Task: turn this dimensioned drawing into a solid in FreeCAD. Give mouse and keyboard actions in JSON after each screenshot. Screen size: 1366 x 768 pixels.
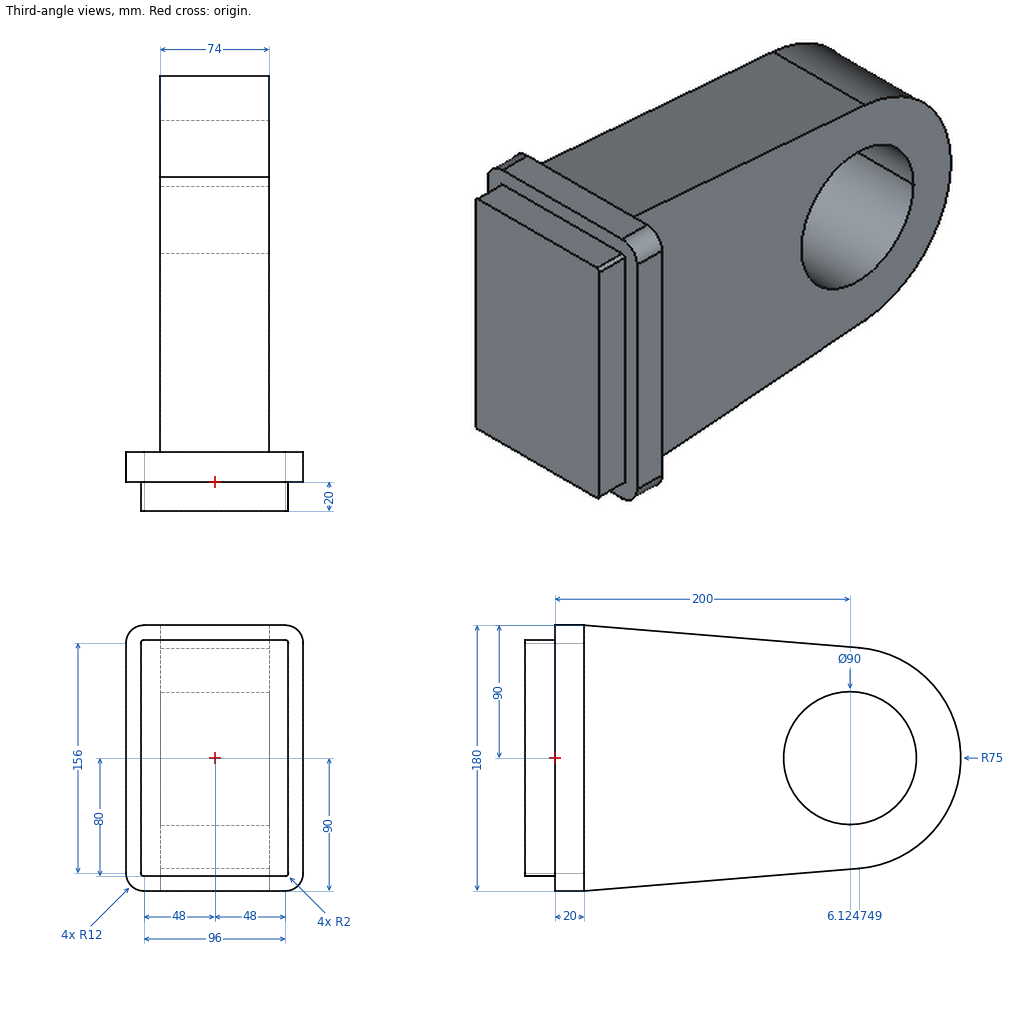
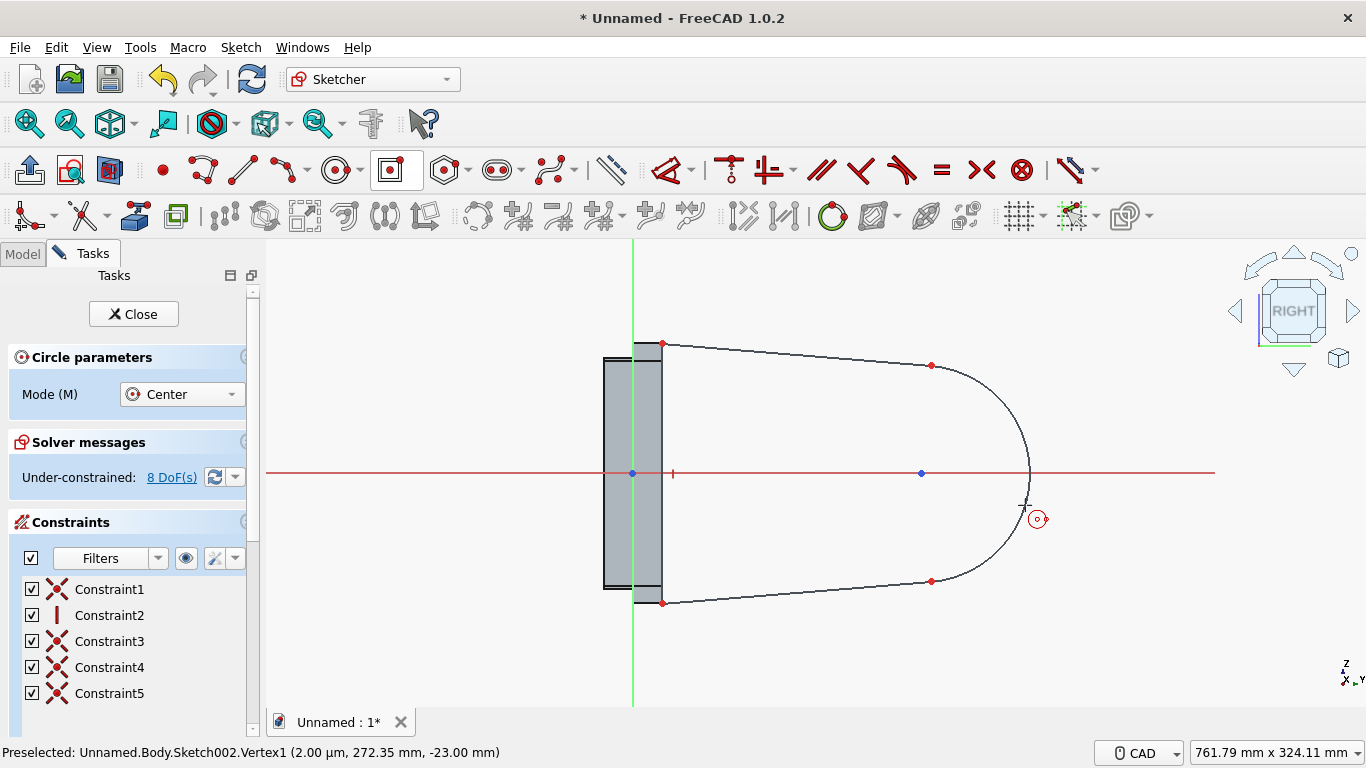
{"action": "left_click", "coordinate": [922, 473]}
{"action": "mouse_move", "coordinate": [968, 427]}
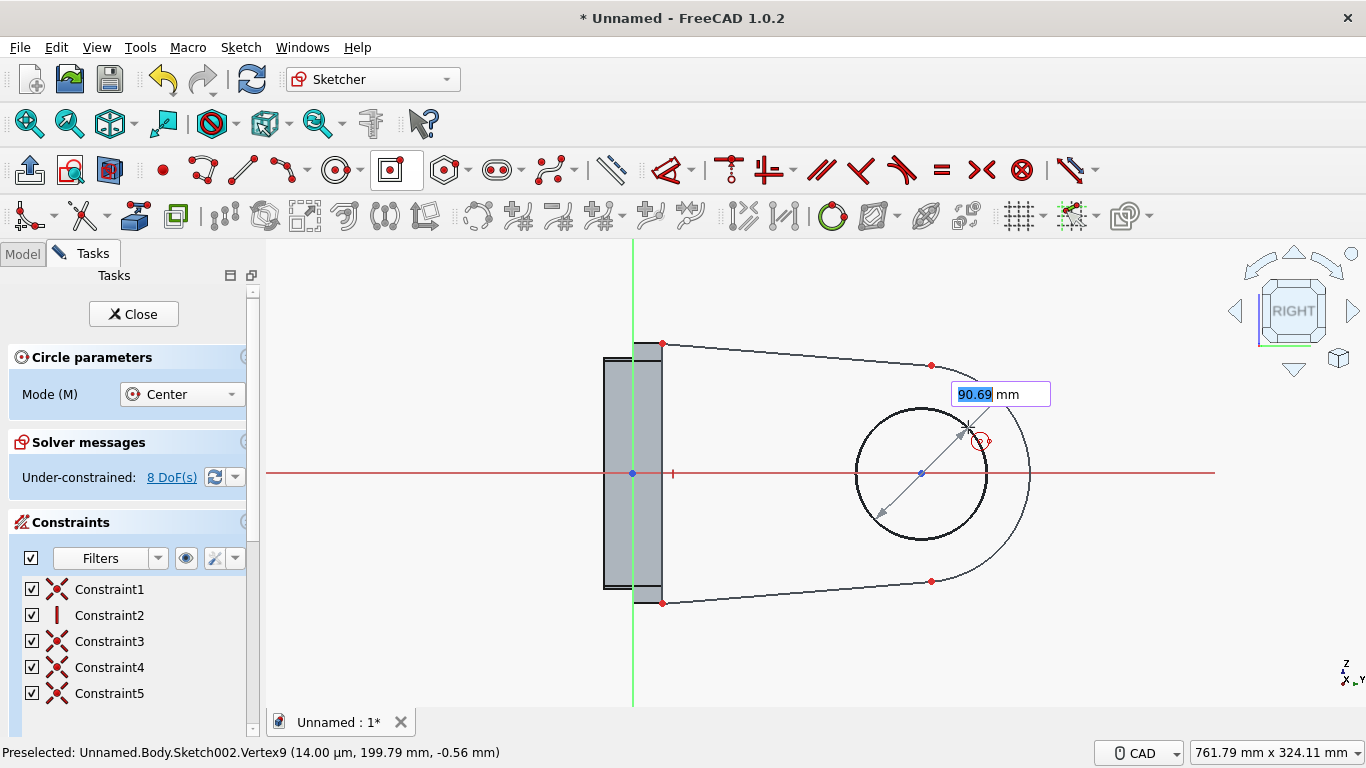
{"action": "type", "text": "90"}
{"action": "key", "text": "Return"}
{"action": "key", "text": "Escape"}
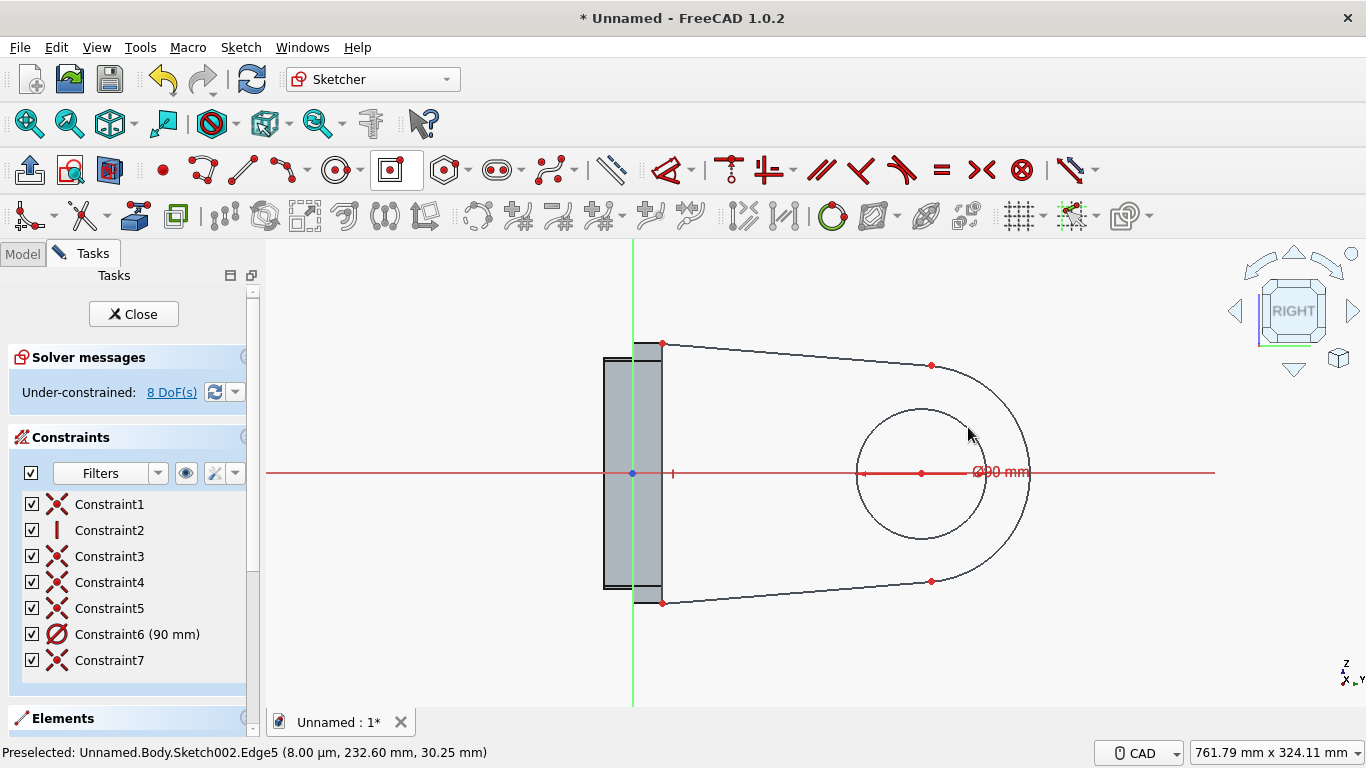
{"action": "left_click", "coordinate": [921, 474]}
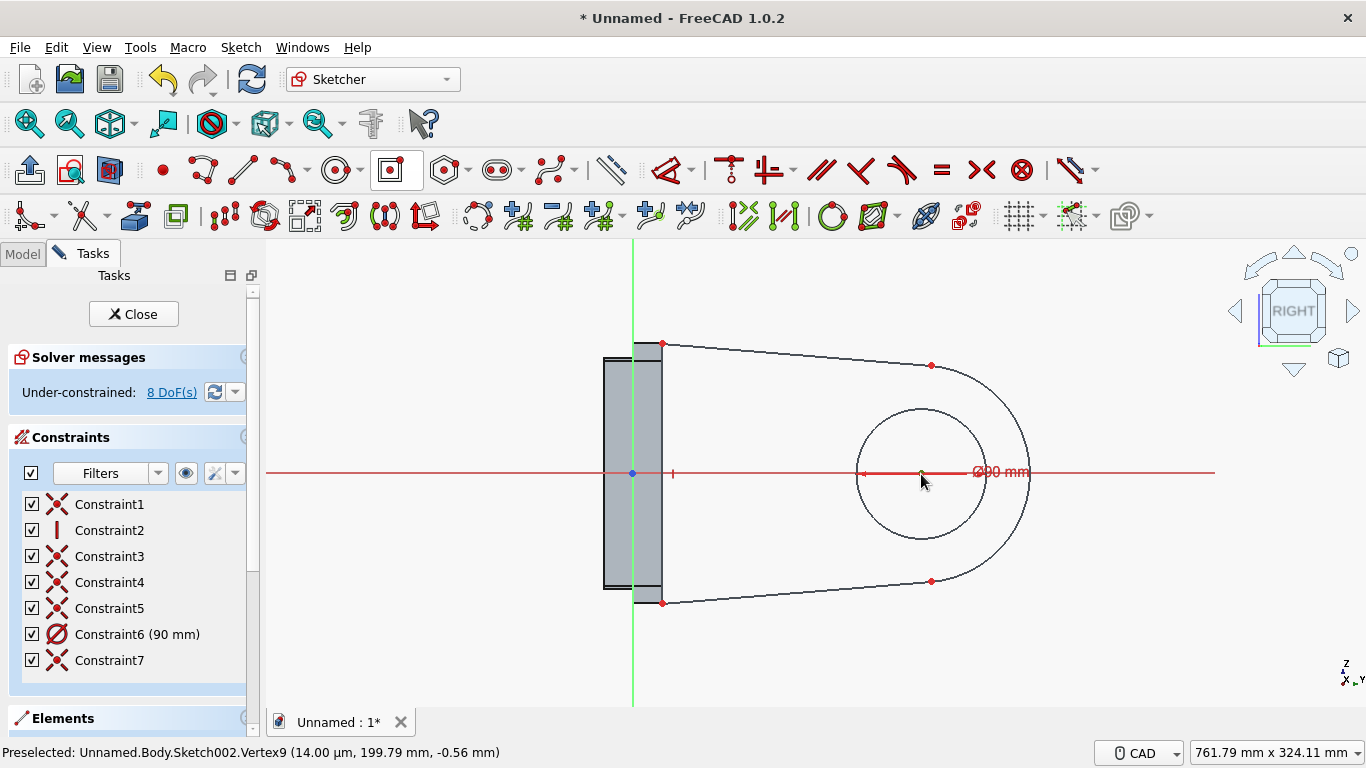
{"action": "left_click", "coordinate": [359, 473]}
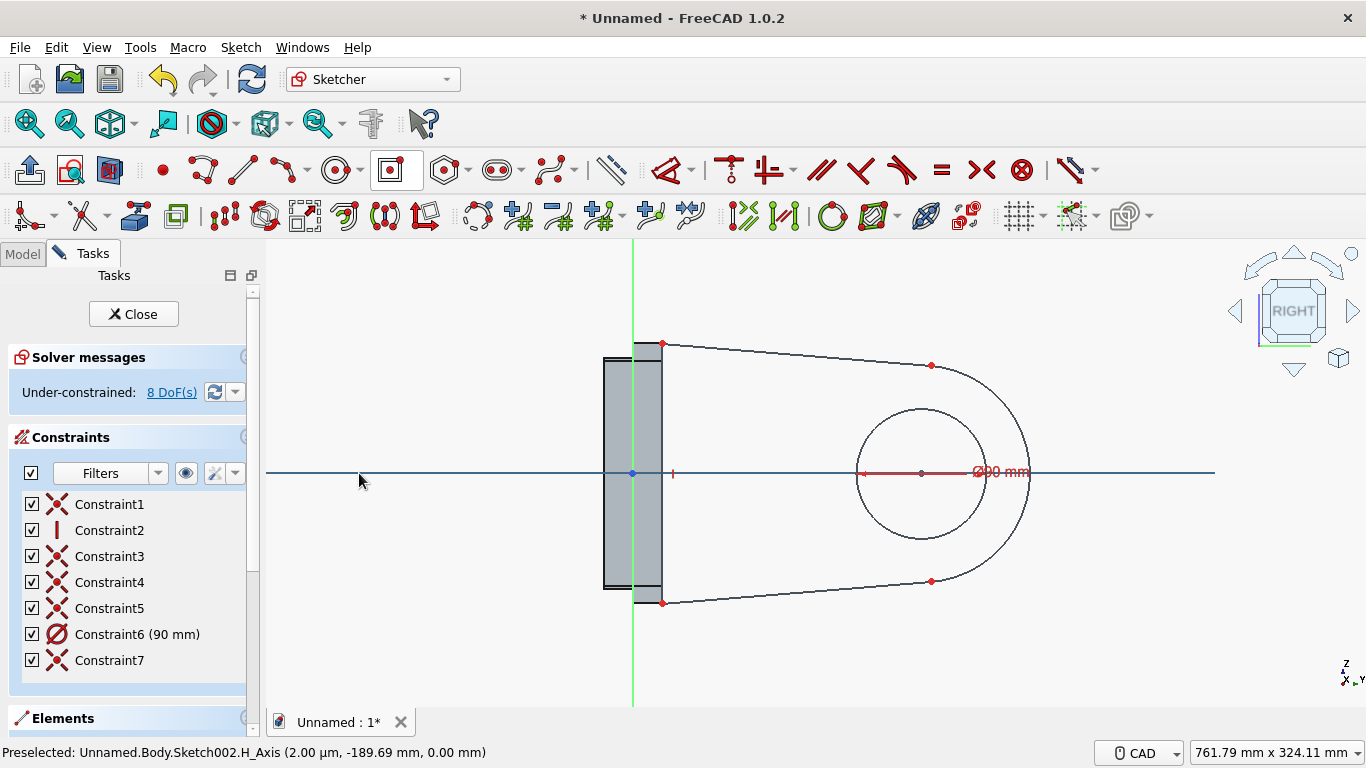
{"action": "left_click", "coordinate": [730, 170]}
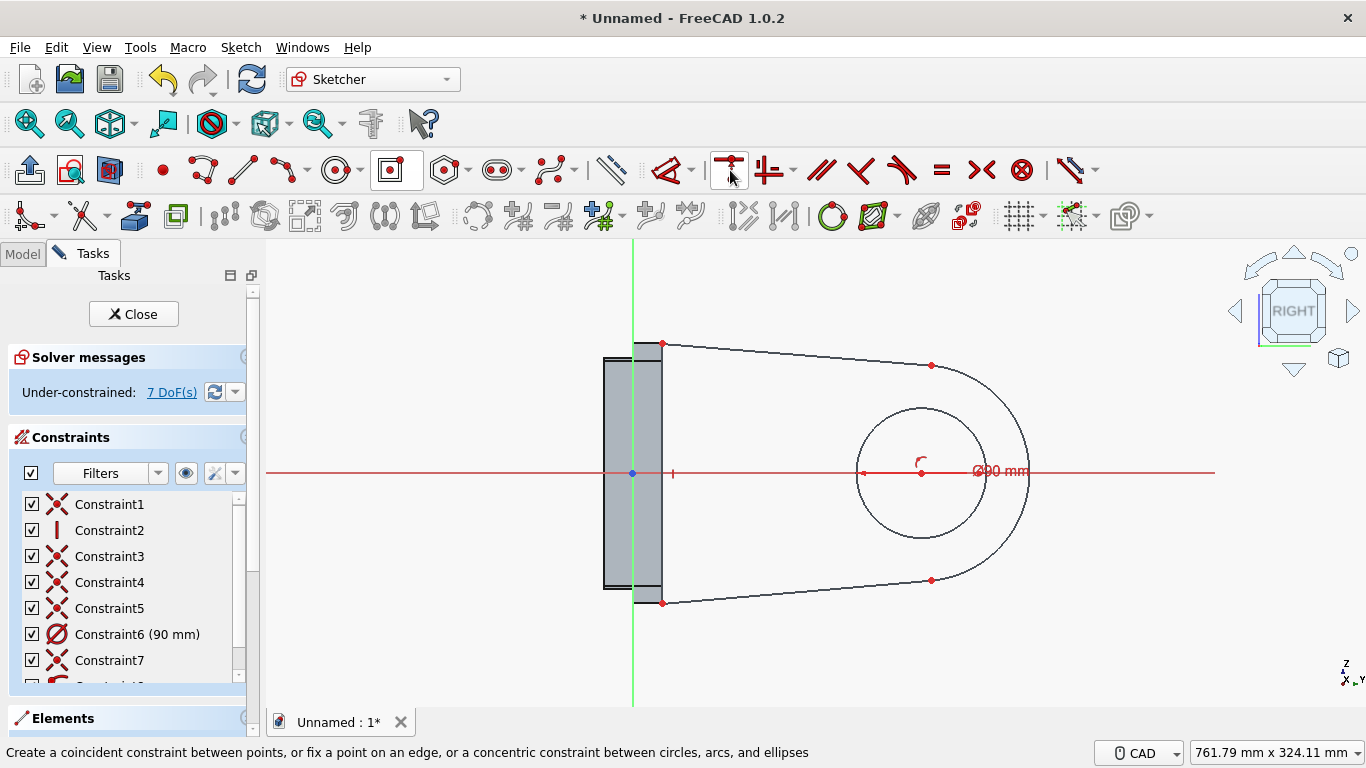
{"action": "key", "text": "d"}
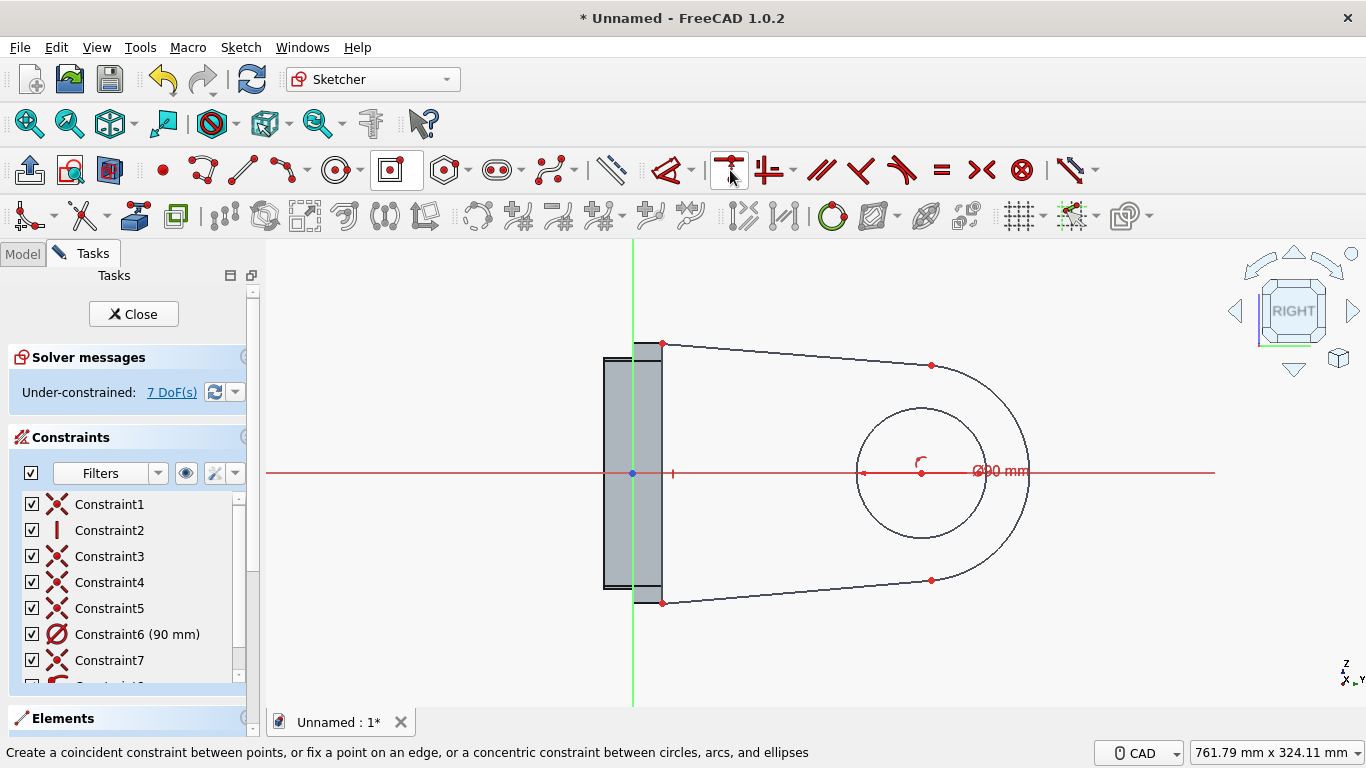
{"action": "left_click", "coordinate": [1011, 534]}
{"action": "left_click", "coordinate": [1037, 552]}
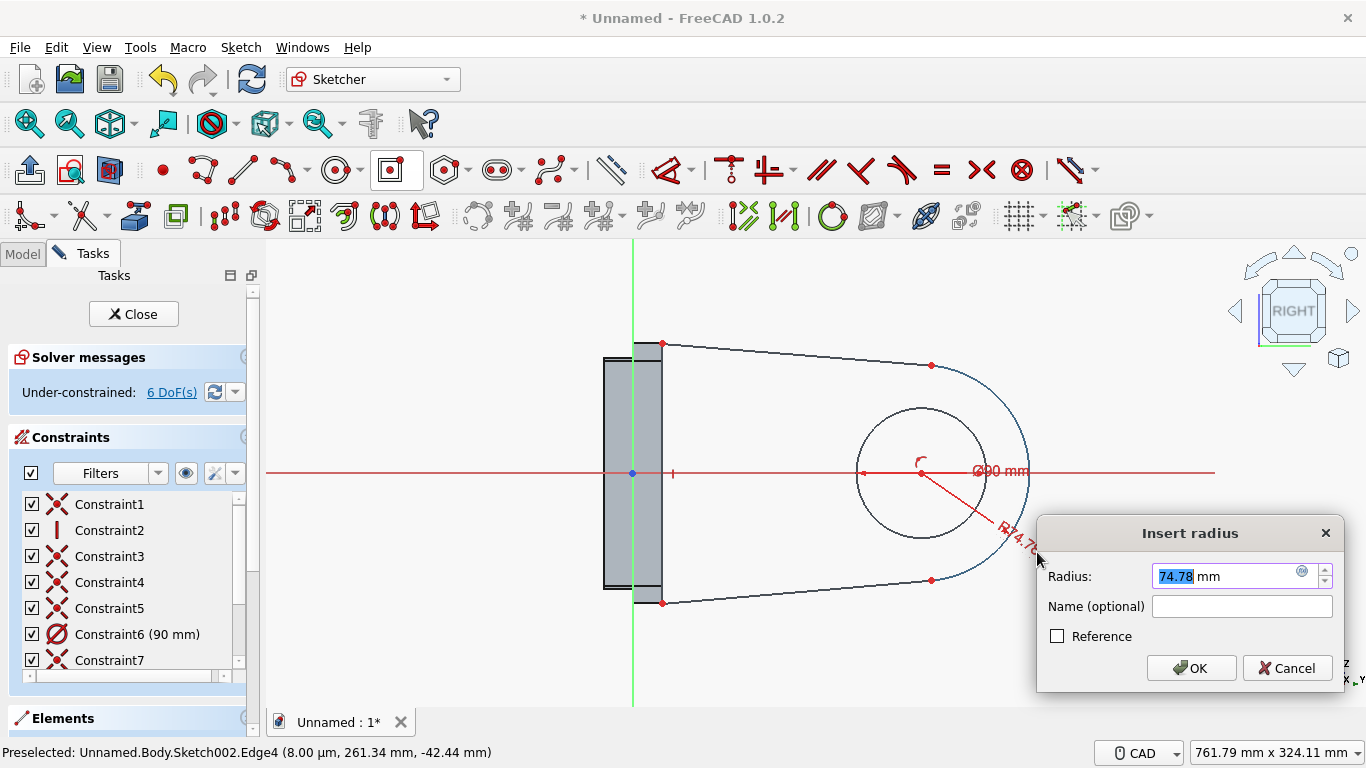
{"action": "type", "text": "75"}
{"action": "key", "text": "Return"}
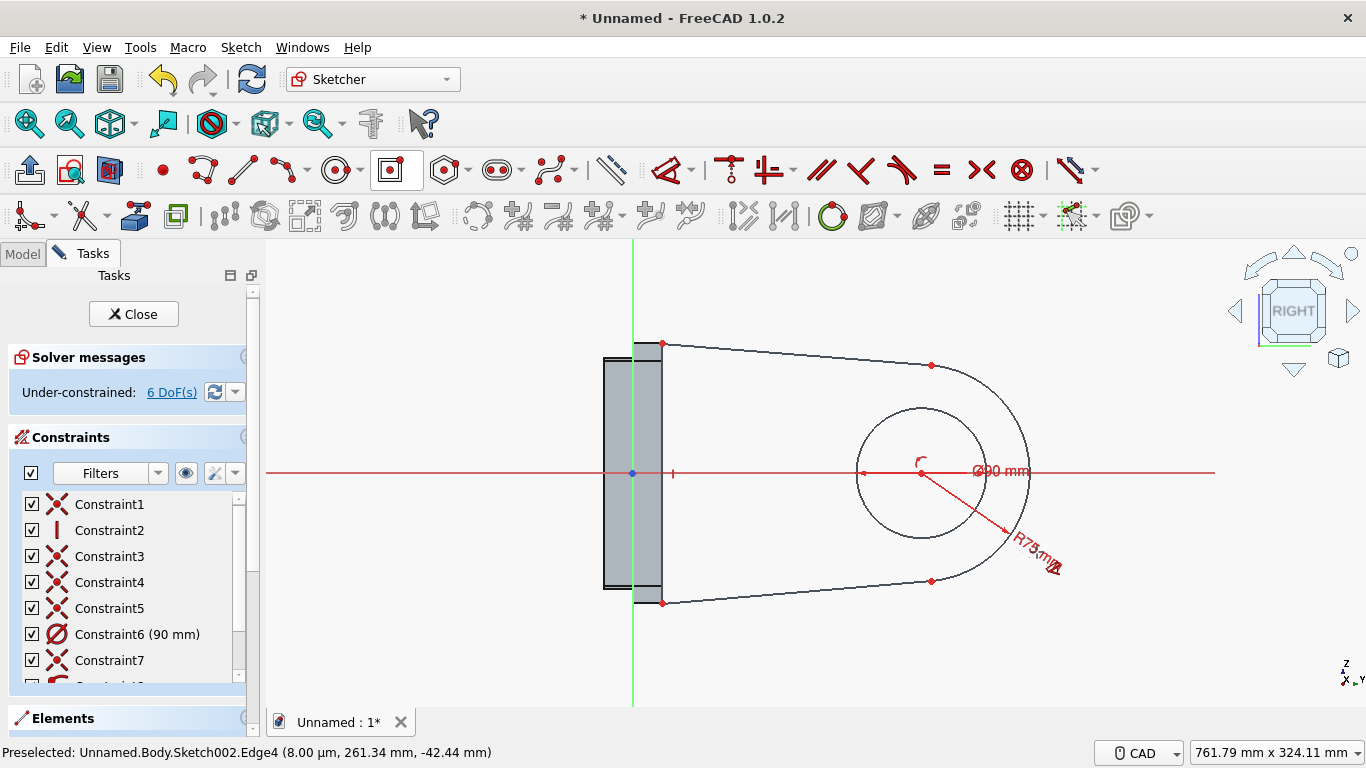
{"action": "left_click", "coordinate": [662, 422]}
{"action": "left_click", "coordinate": [696, 414]}